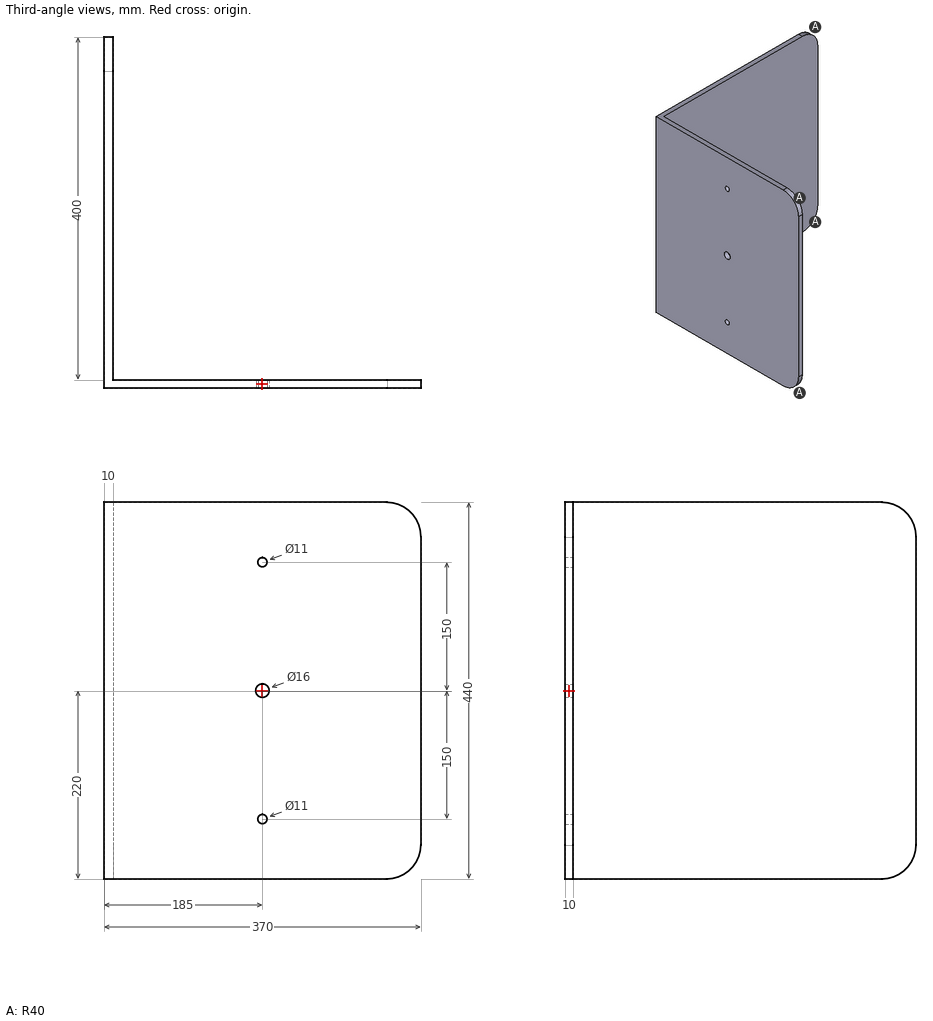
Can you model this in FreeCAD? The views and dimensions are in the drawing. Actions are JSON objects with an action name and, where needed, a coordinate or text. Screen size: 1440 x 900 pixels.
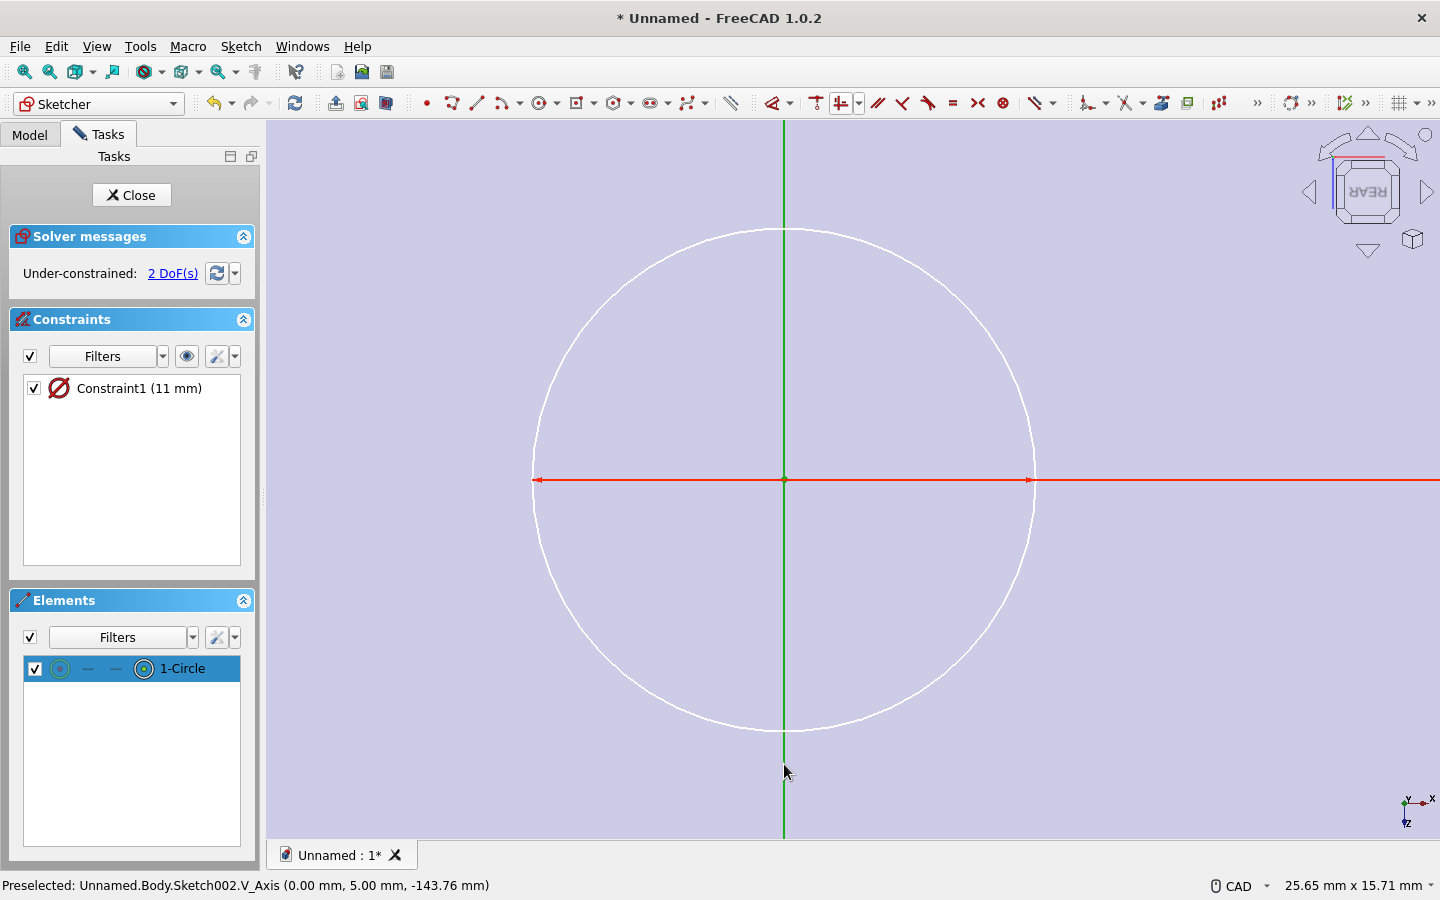
{"action": "left_click", "coordinate": [816, 104]}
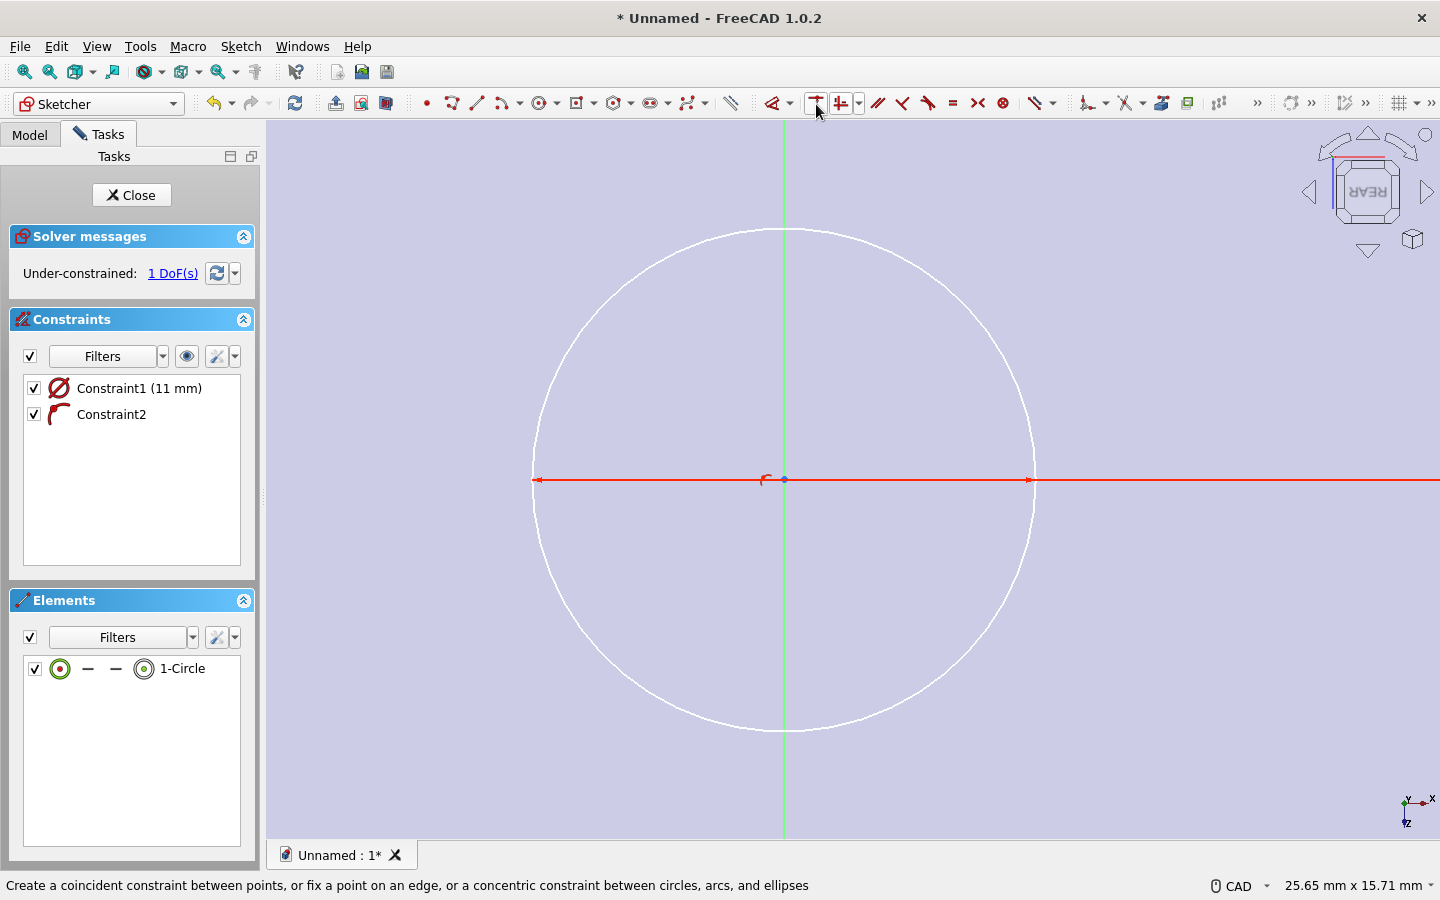
{"action": "left_click", "coordinate": [772, 104]}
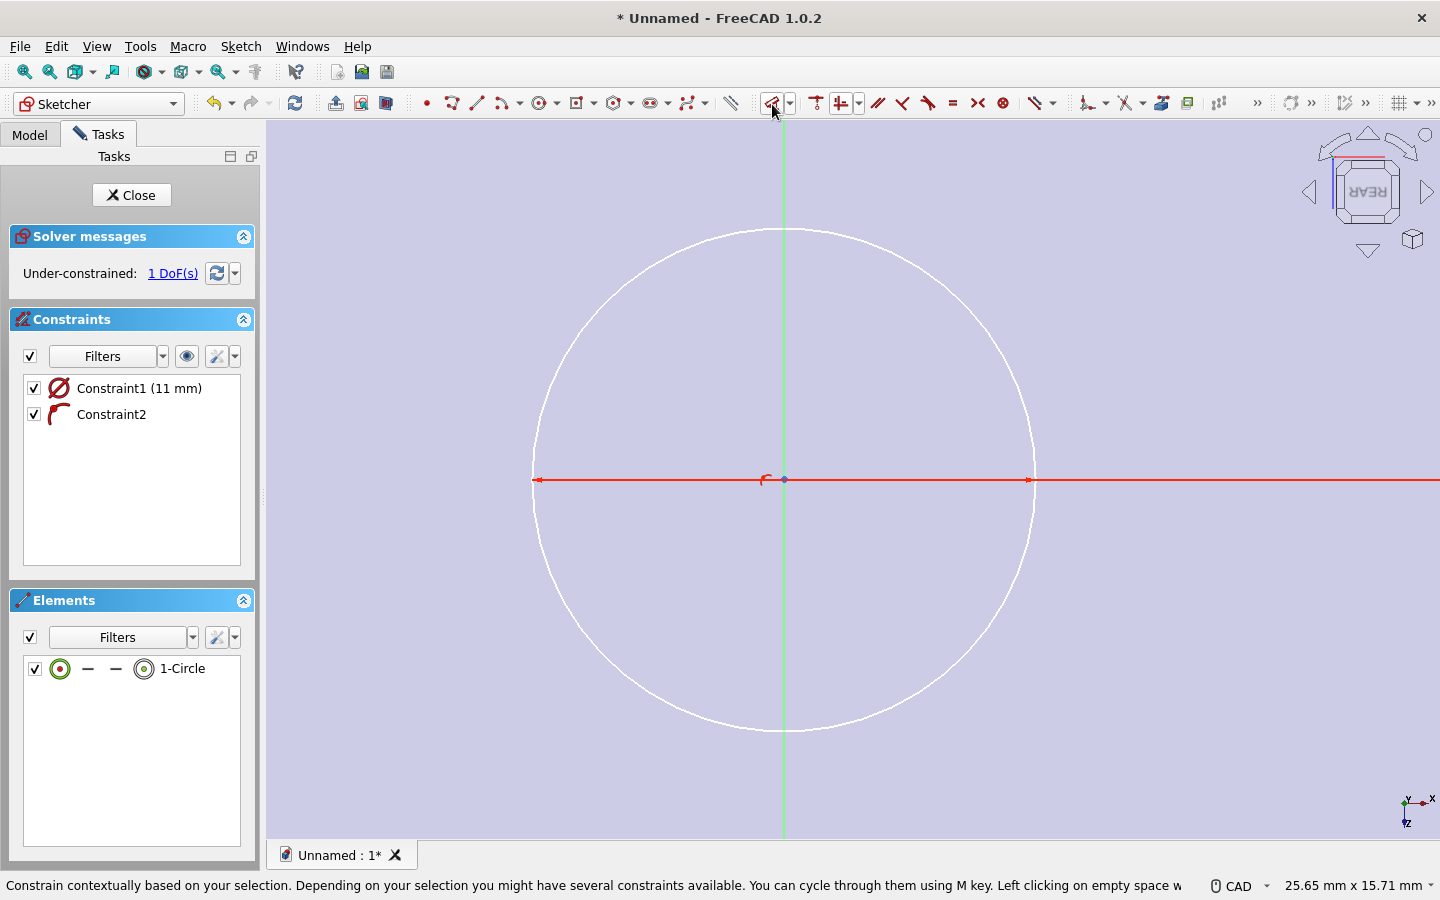
{"action": "left_click", "coordinate": [784, 480]}
{"action": "left_click", "coordinate": [818, 646]}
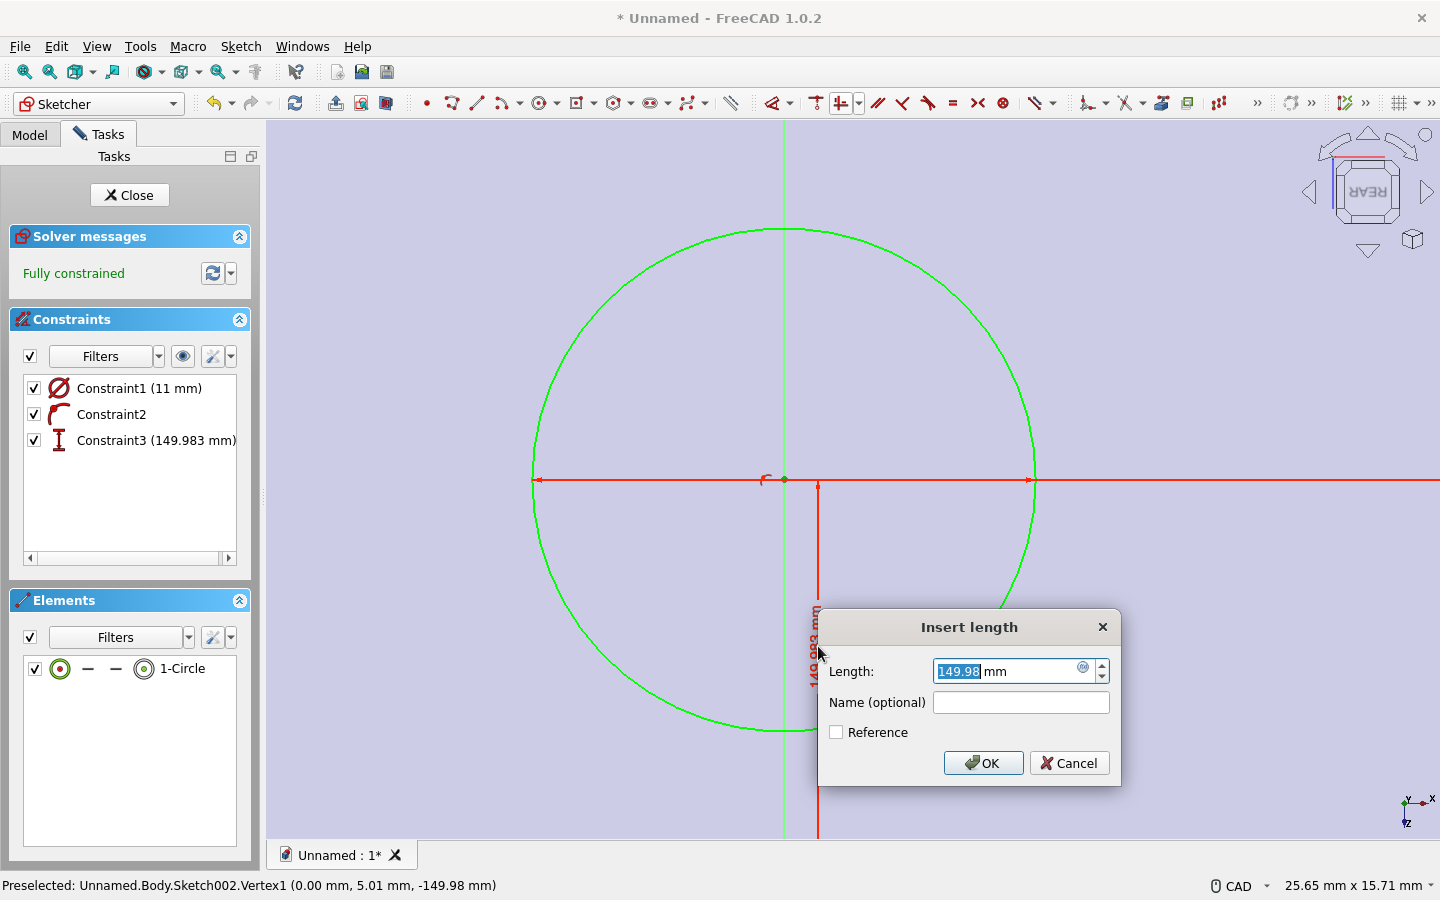
{"action": "type", "text": "150"}
{"action": "key", "text": "Return"}
{"action": "key", "text": "Escape"}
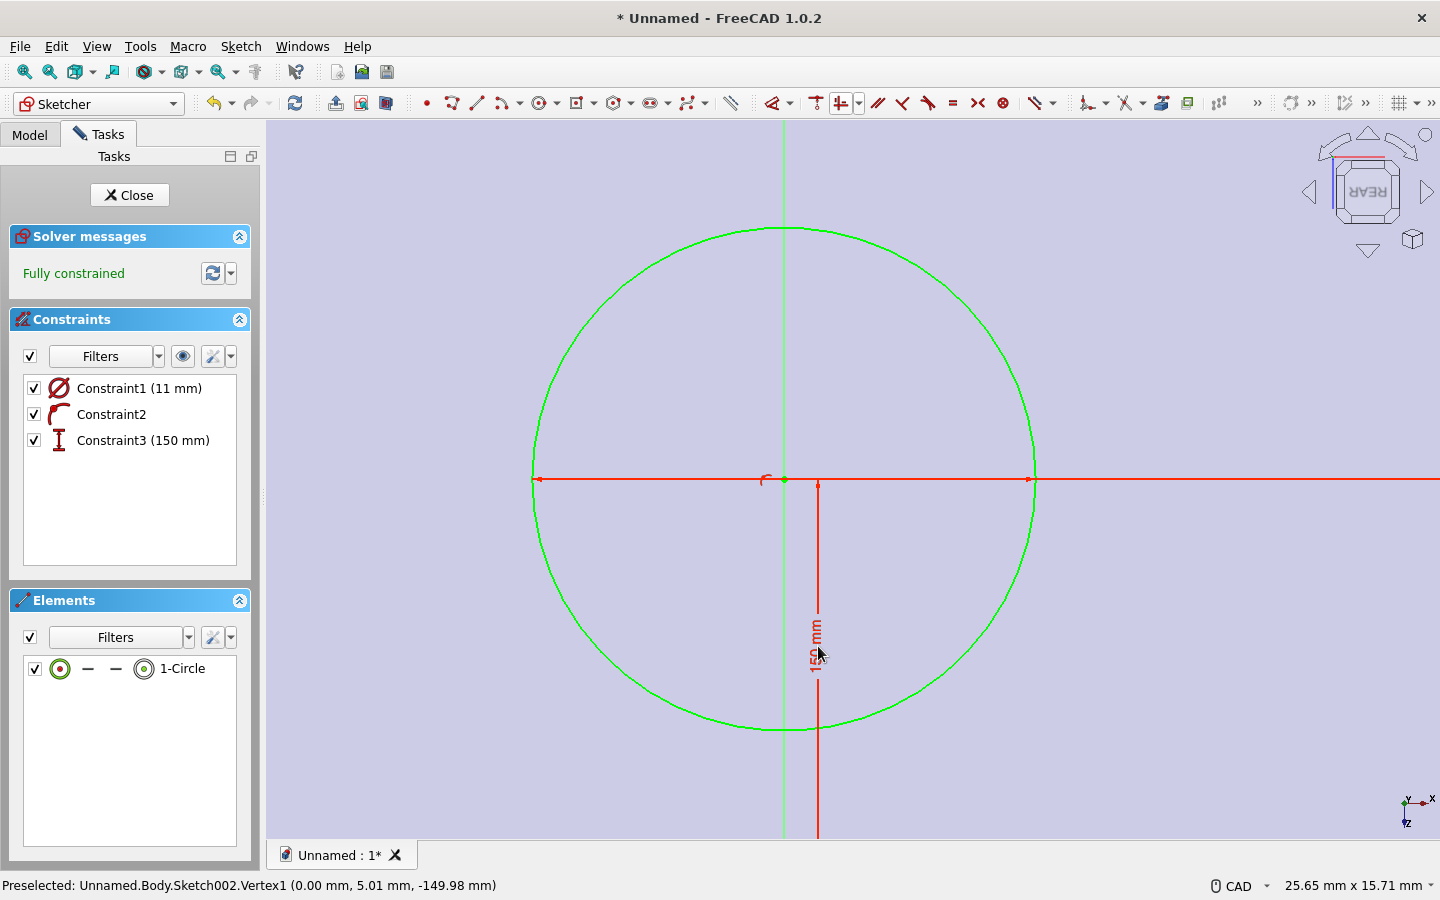
{"action": "left_click", "coordinate": [130, 195]}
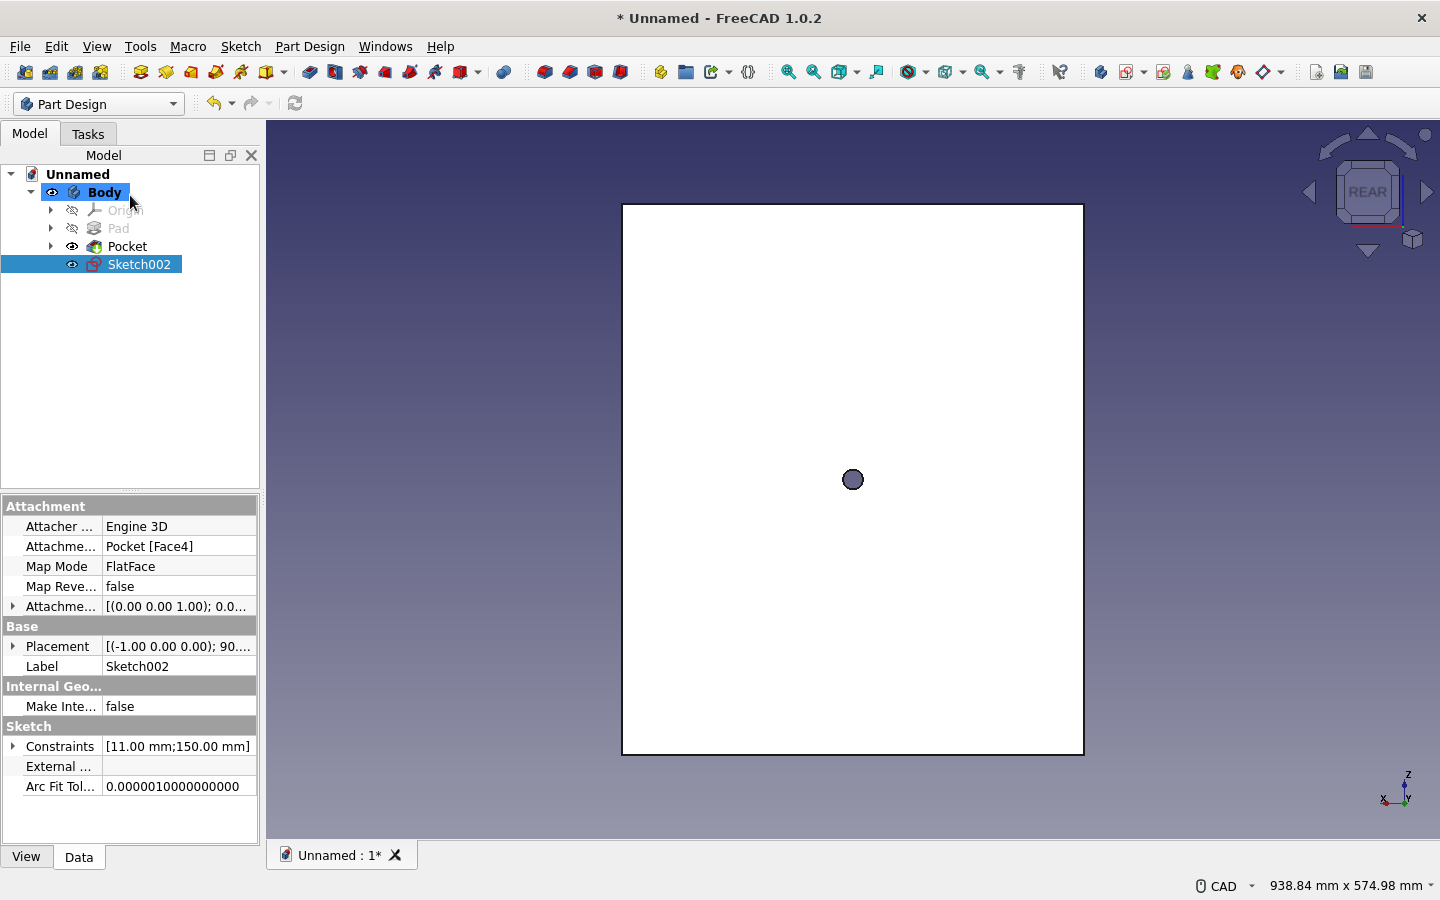
{"action": "left_click", "coordinate": [310, 72]}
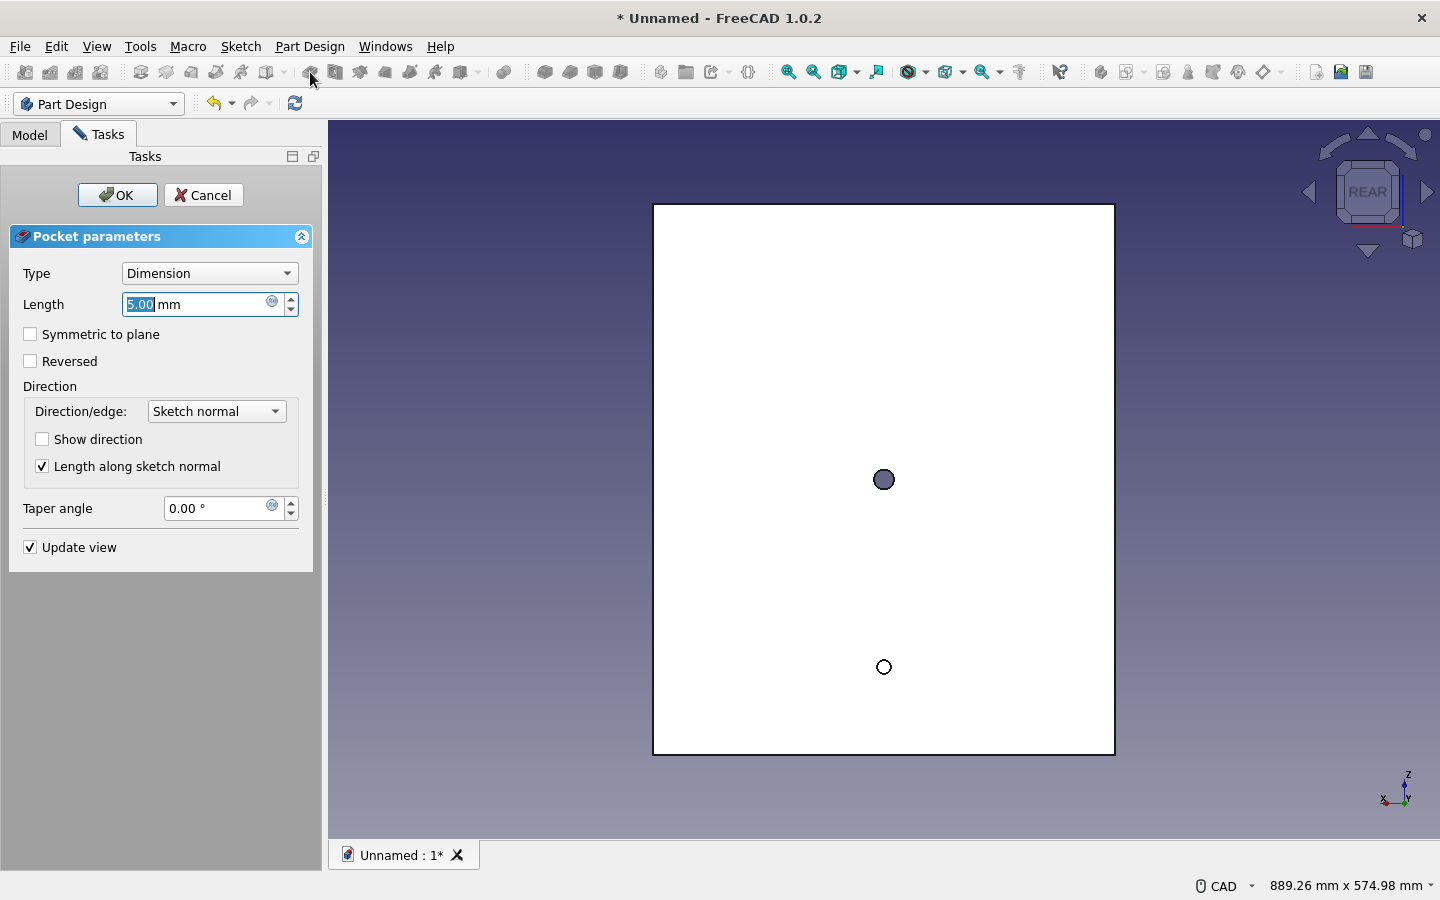
{"action": "left_click", "coordinate": [210, 274]}